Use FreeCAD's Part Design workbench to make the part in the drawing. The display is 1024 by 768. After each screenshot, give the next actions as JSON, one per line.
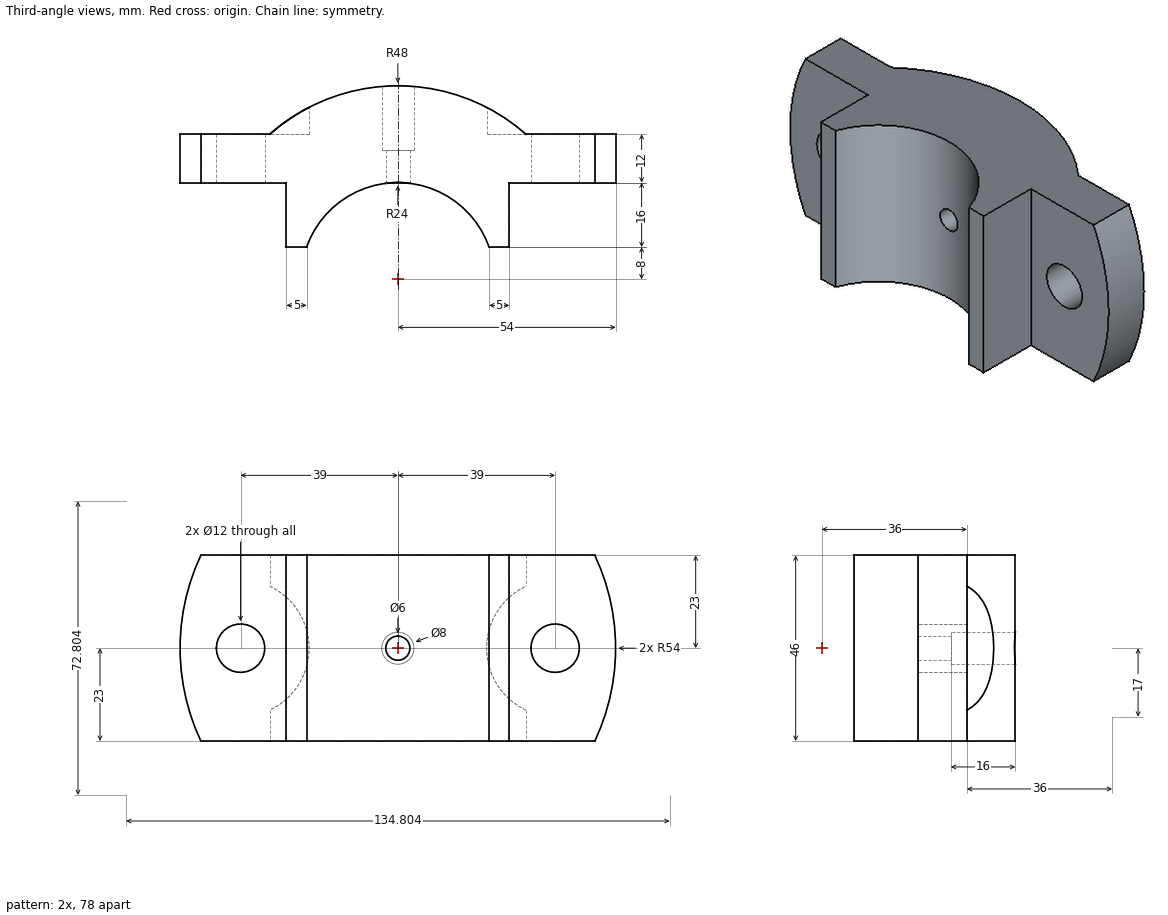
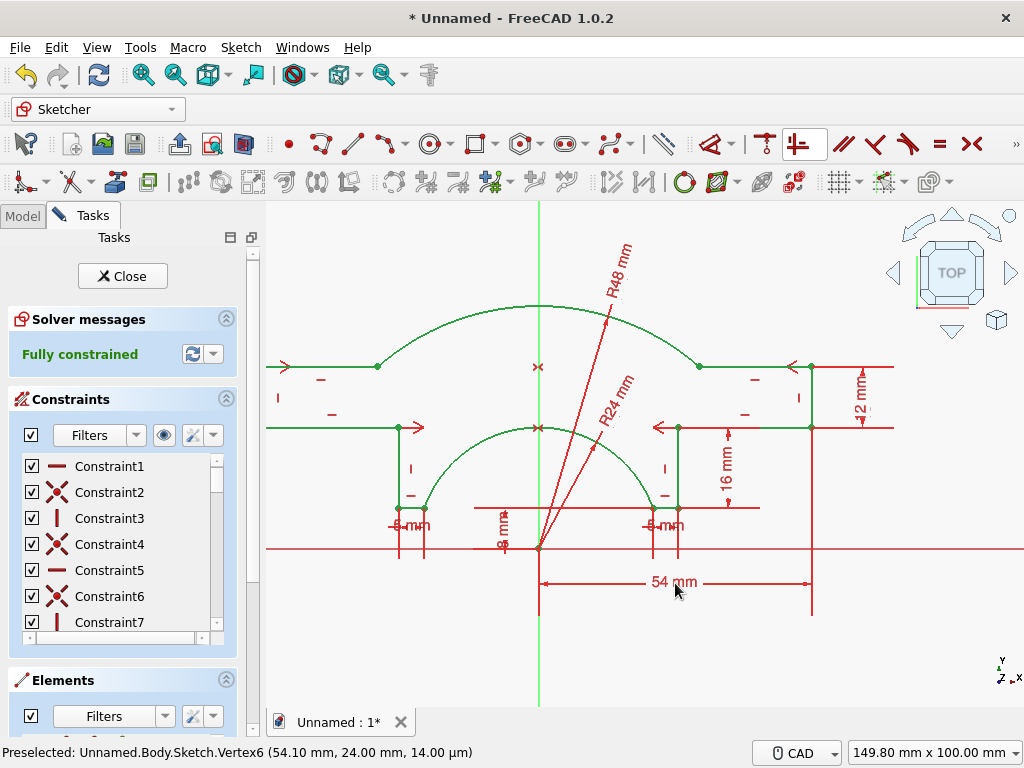
{"action": "left_click", "coordinate": [123, 276]}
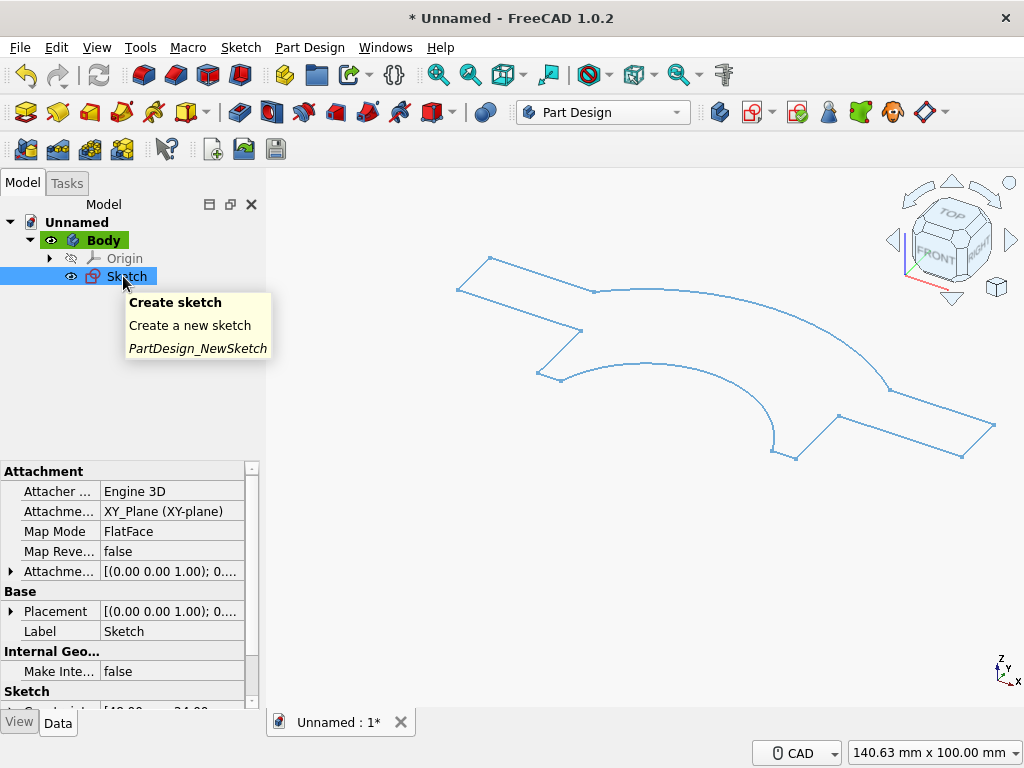
{"action": "left_click", "coordinate": [26, 112]}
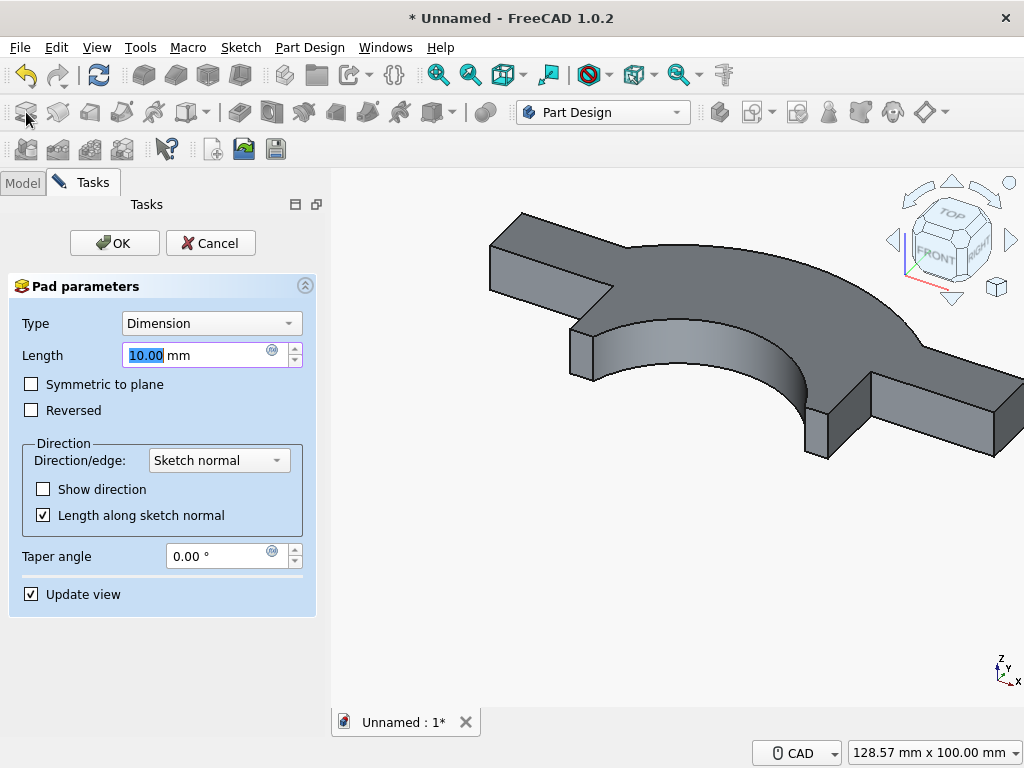
{"action": "type", "text": "46"}
{"action": "key", "text": "Tab"}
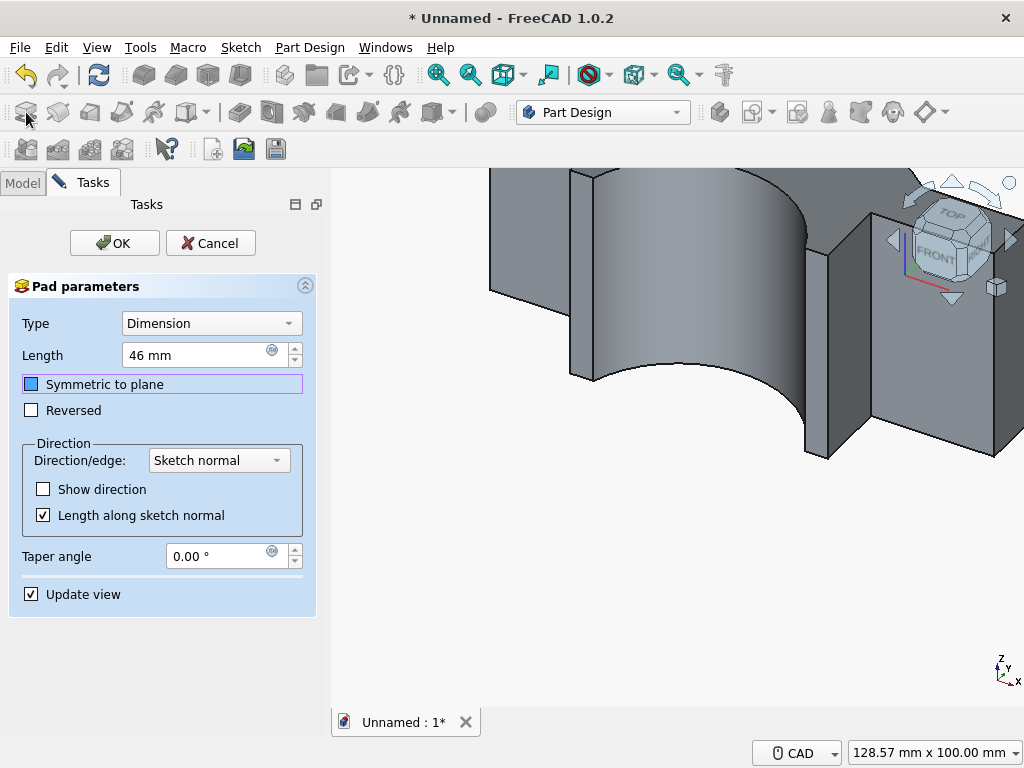
{"action": "left_click", "coordinate": [30, 384]}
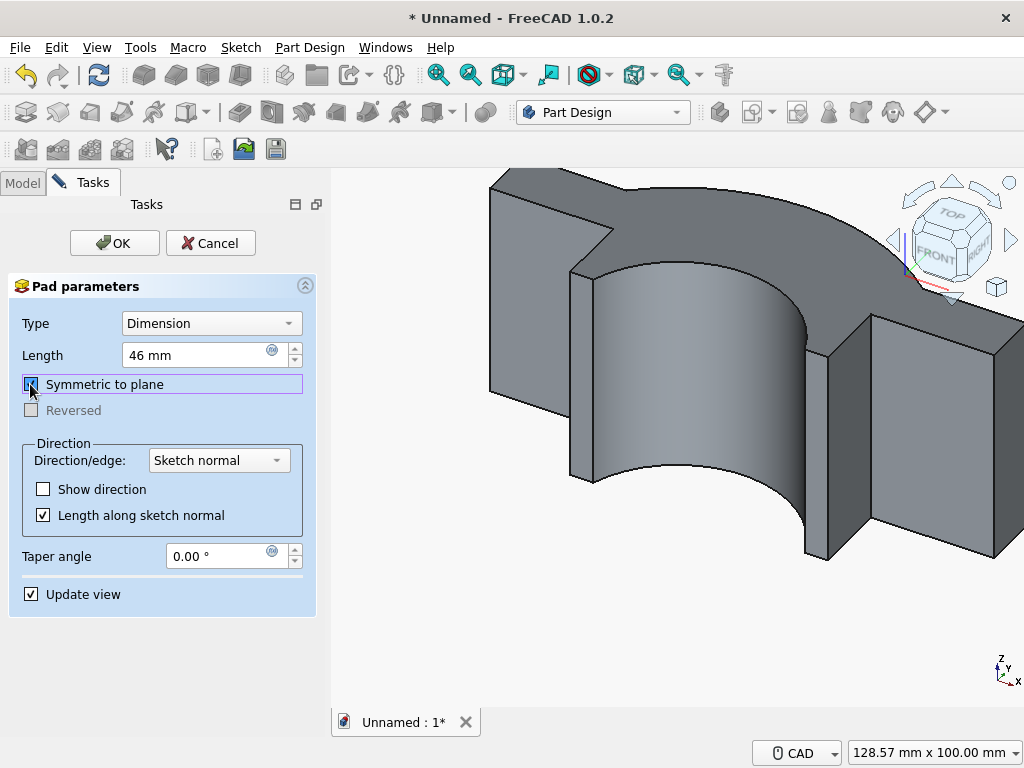
{"action": "left_click", "coordinate": [115, 243]}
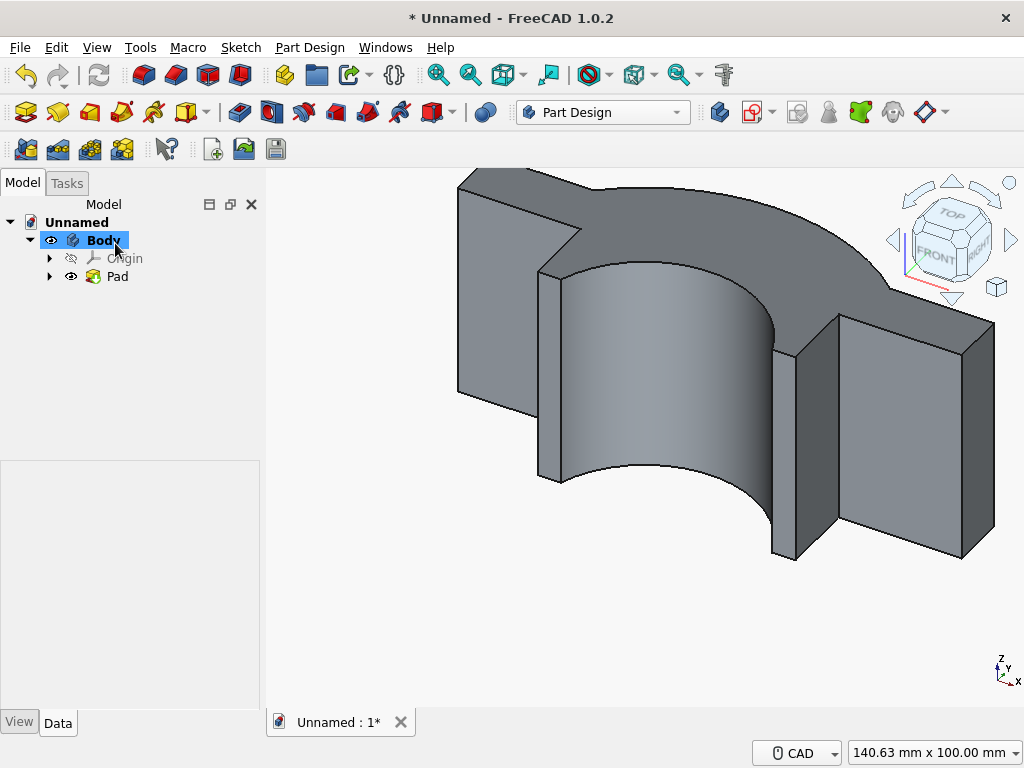
{"action": "key", "text": "v f"}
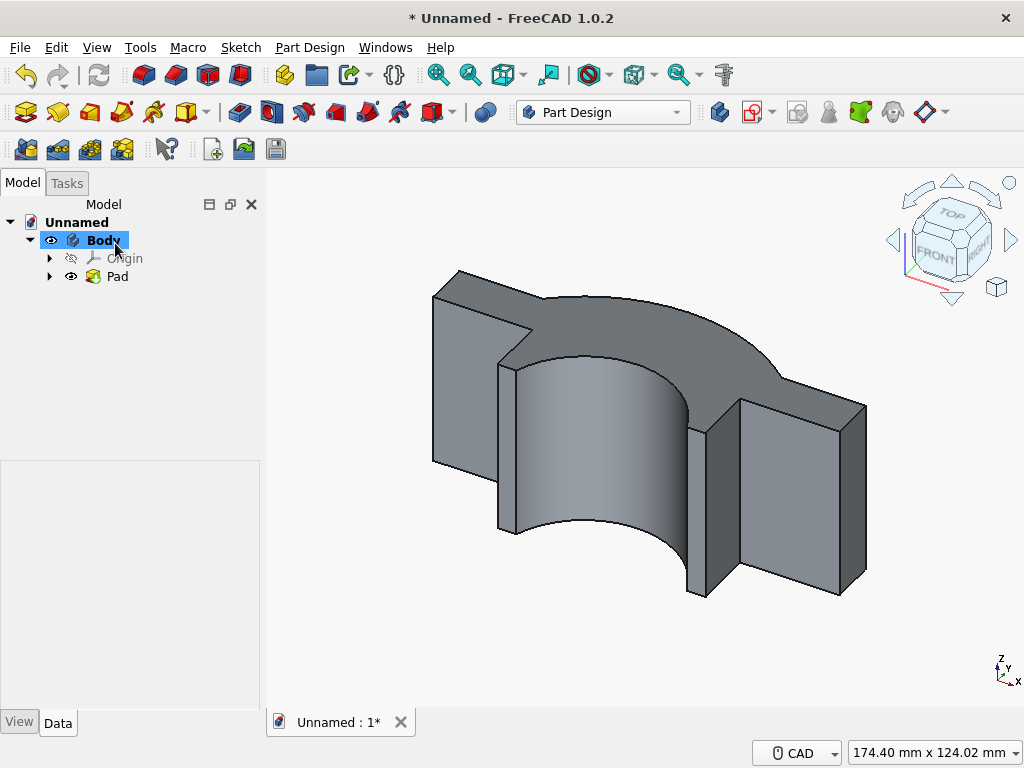
{"action": "key", "text": "4"}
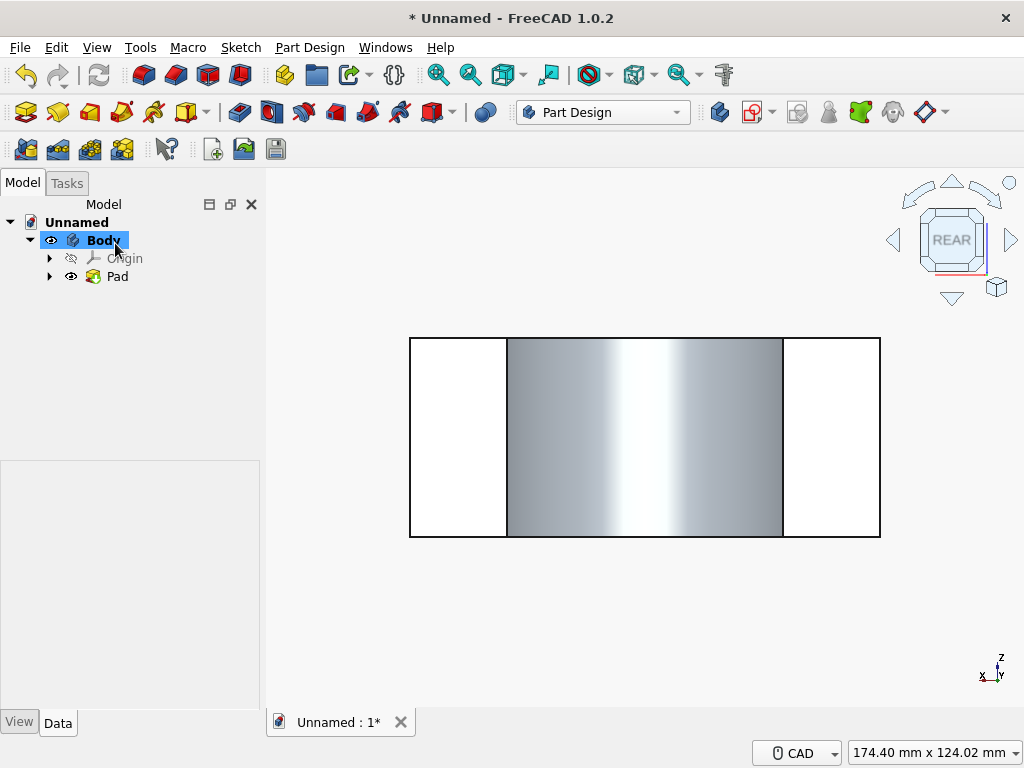
{"action": "left_click", "coordinate": [831, 408]}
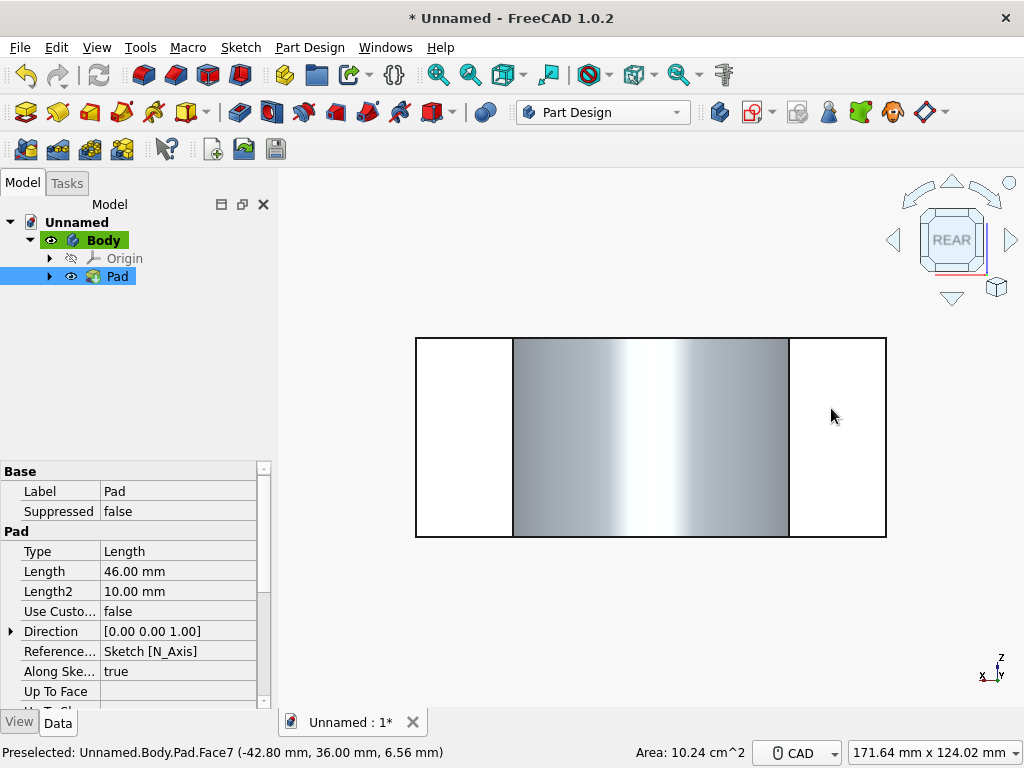
{"action": "left_click", "coordinate": [752, 112]}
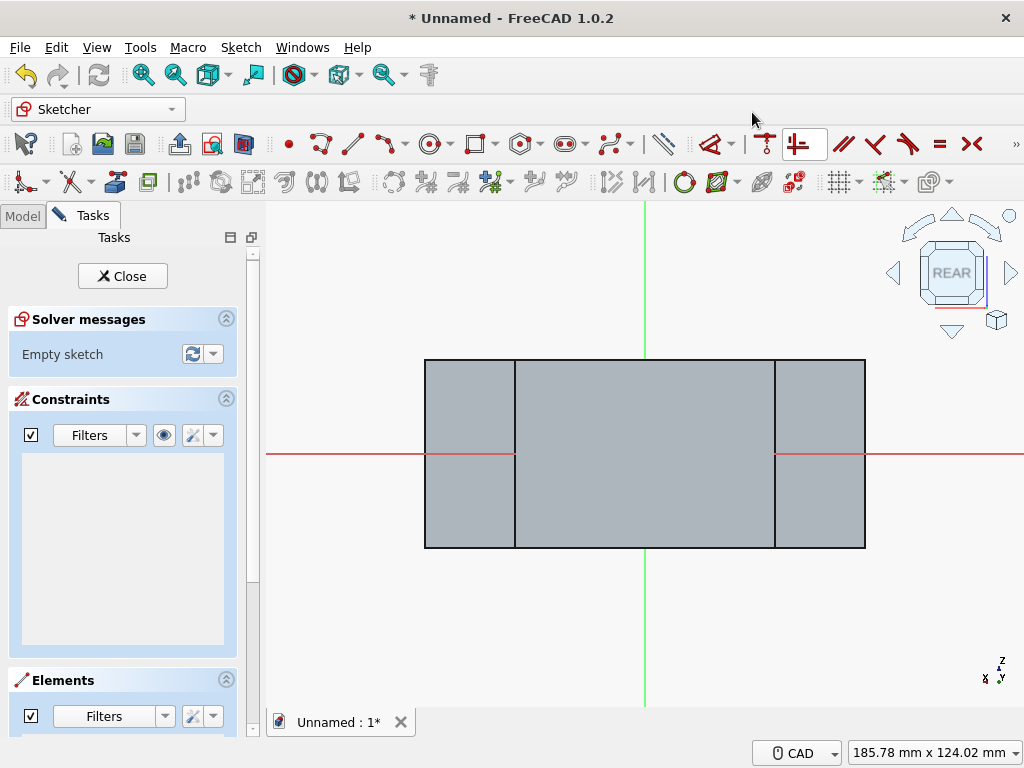
{"action": "left_click", "coordinate": [430, 144]}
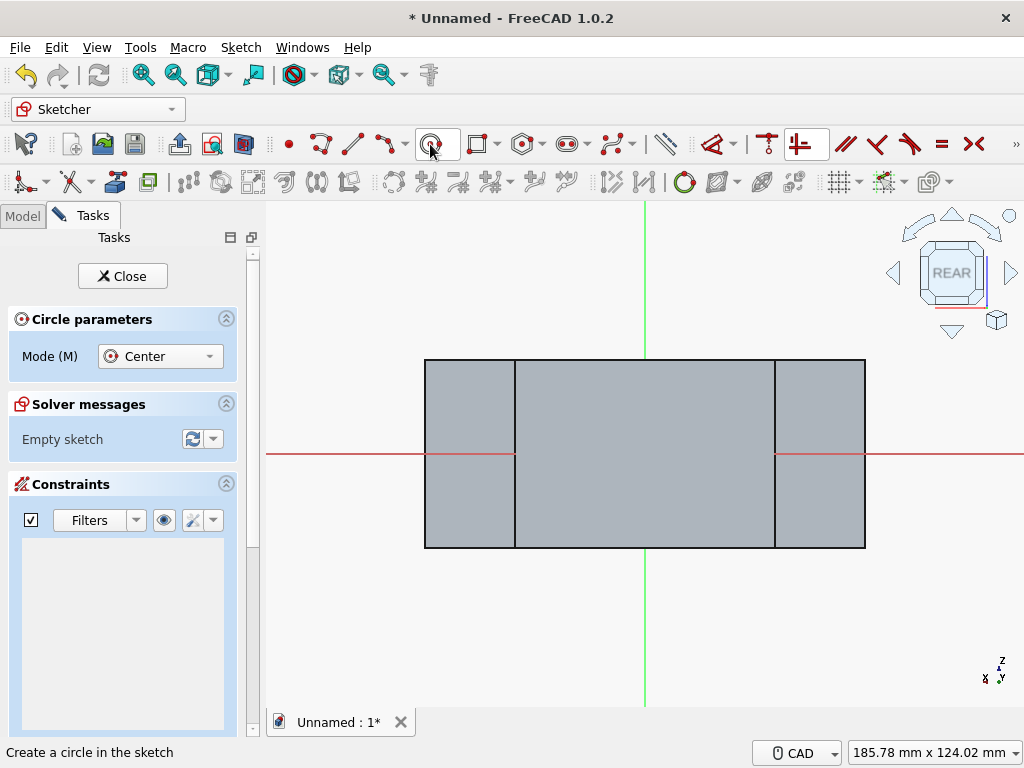
{"action": "left_click", "coordinate": [804, 454]}
{"action": "mouse_move", "coordinate": [821, 437]}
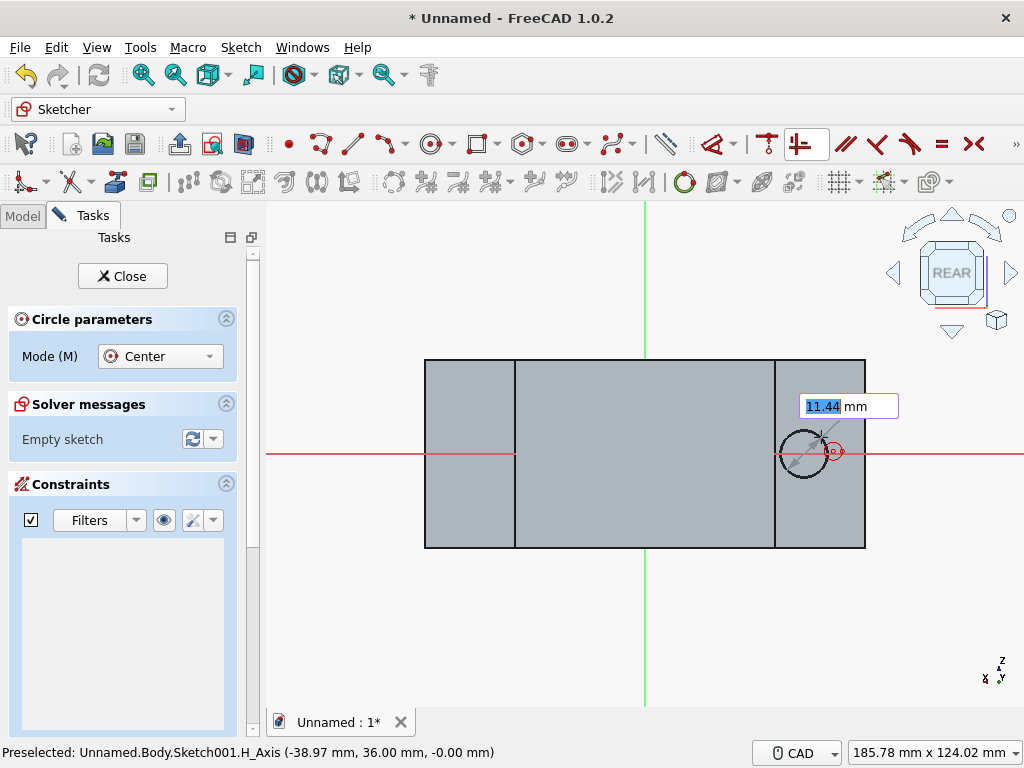
{"action": "type", "text": "12"}
{"action": "key", "text": "Return"}